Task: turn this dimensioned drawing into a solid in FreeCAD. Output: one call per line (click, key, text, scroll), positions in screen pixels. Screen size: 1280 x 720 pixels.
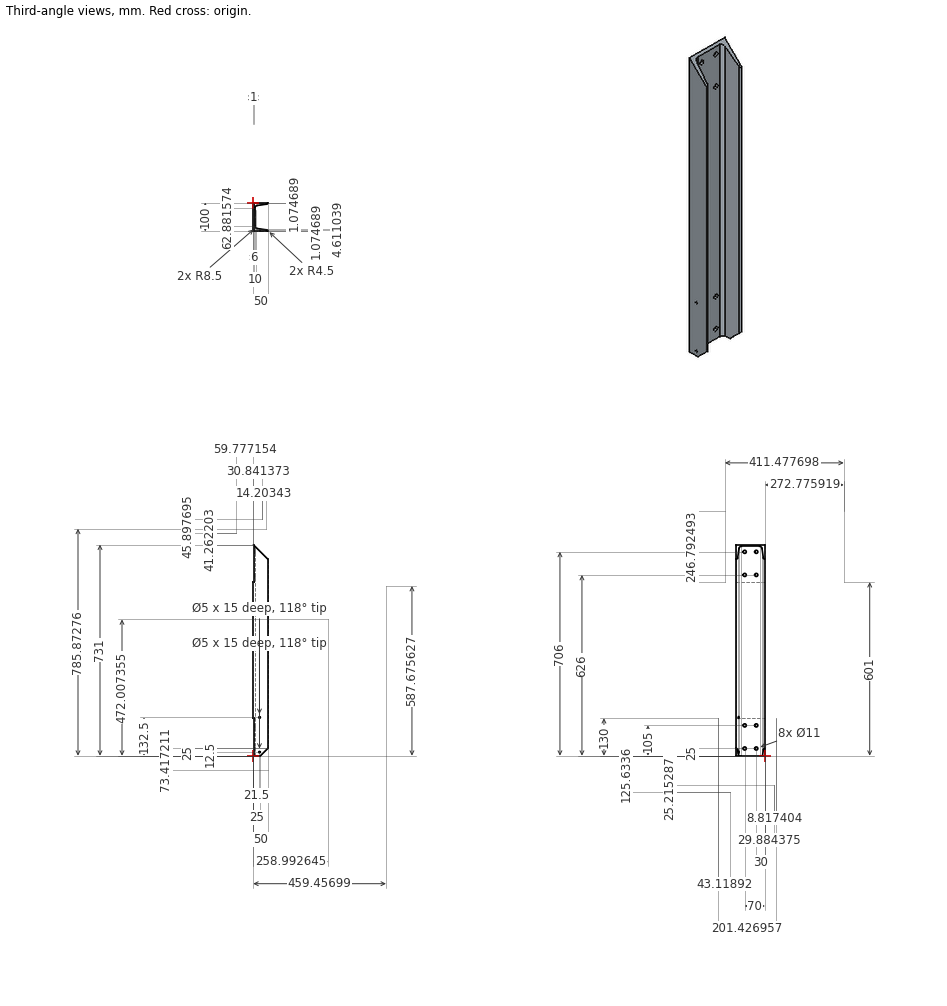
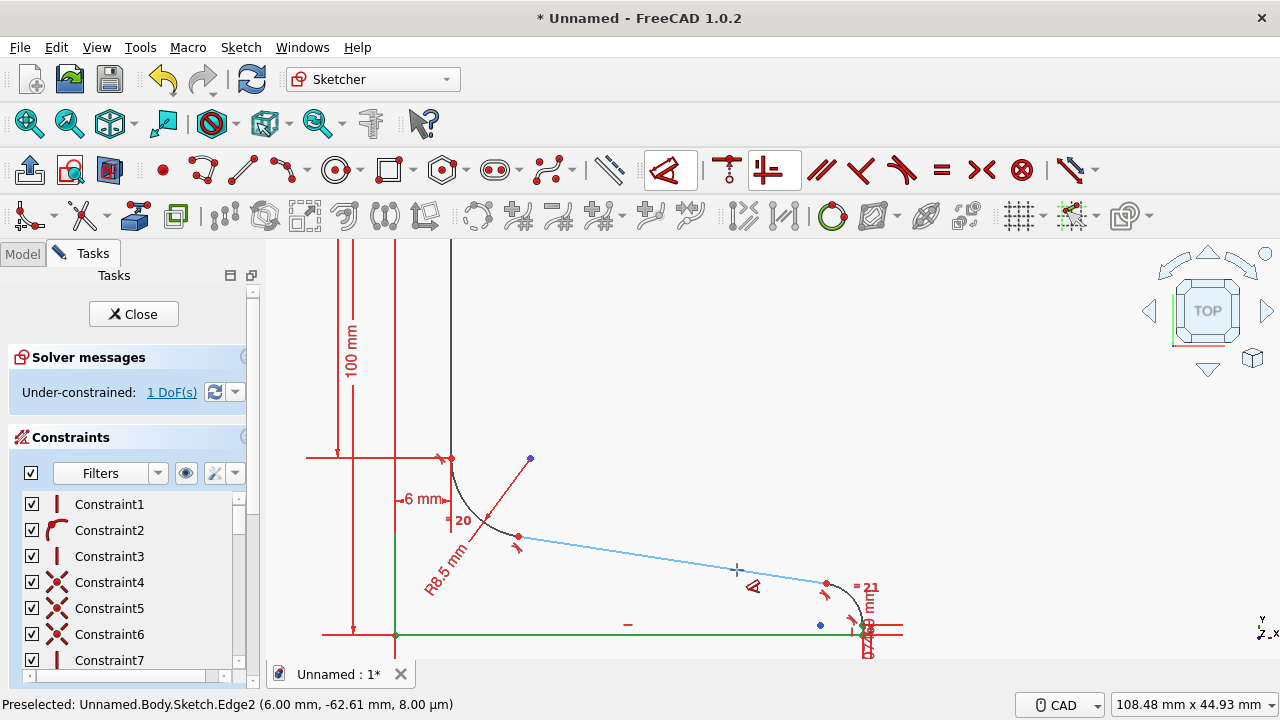
click(734, 570)
click(861, 560)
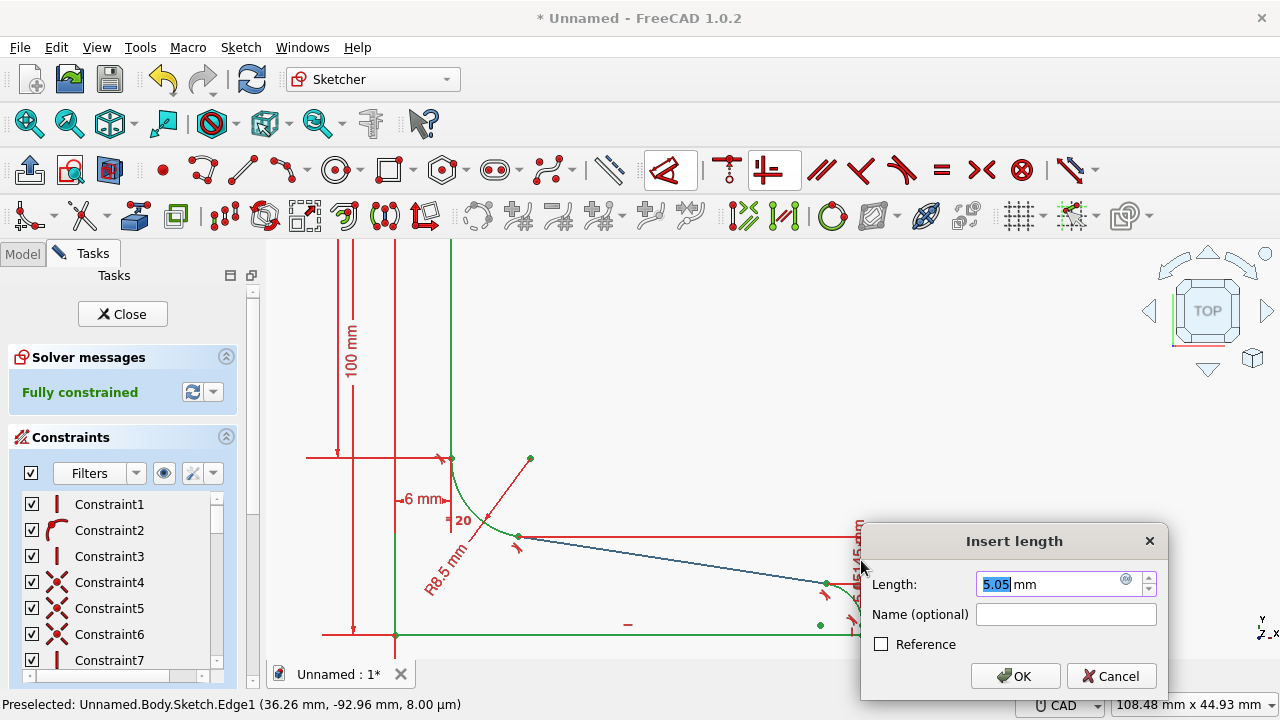
text(4.611039)
key(Return)
key(Escape)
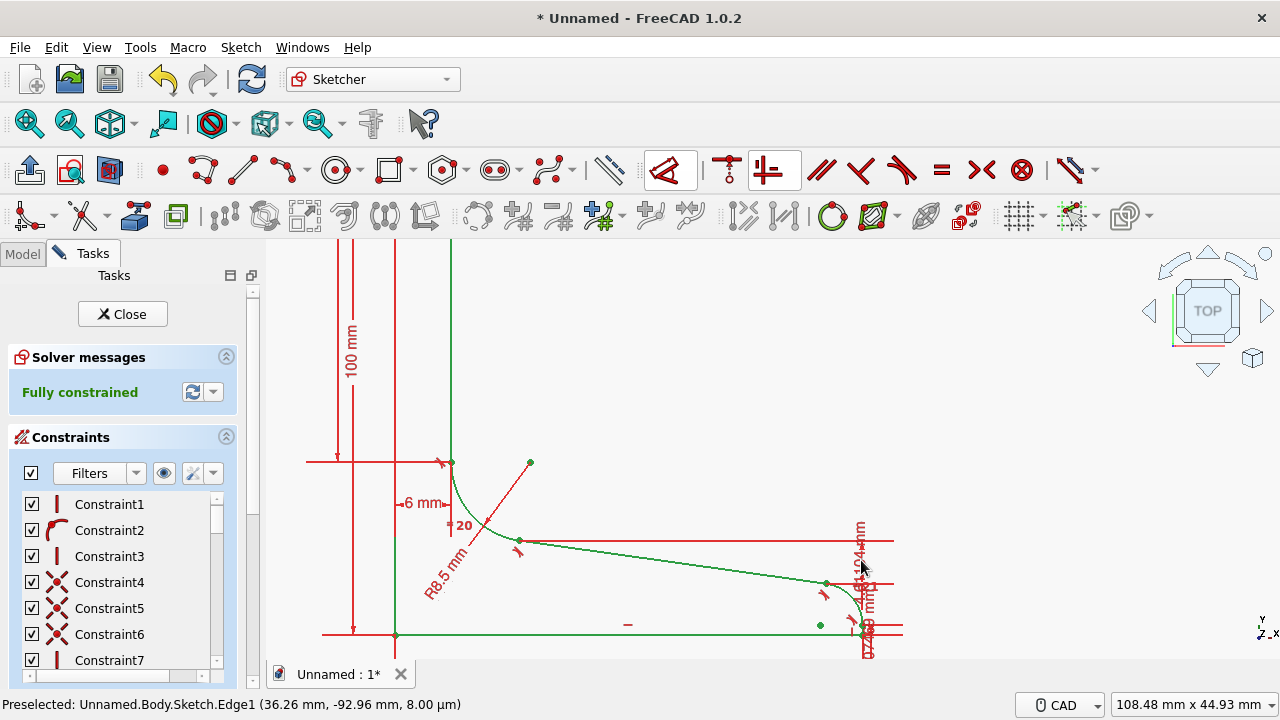
click(123, 314)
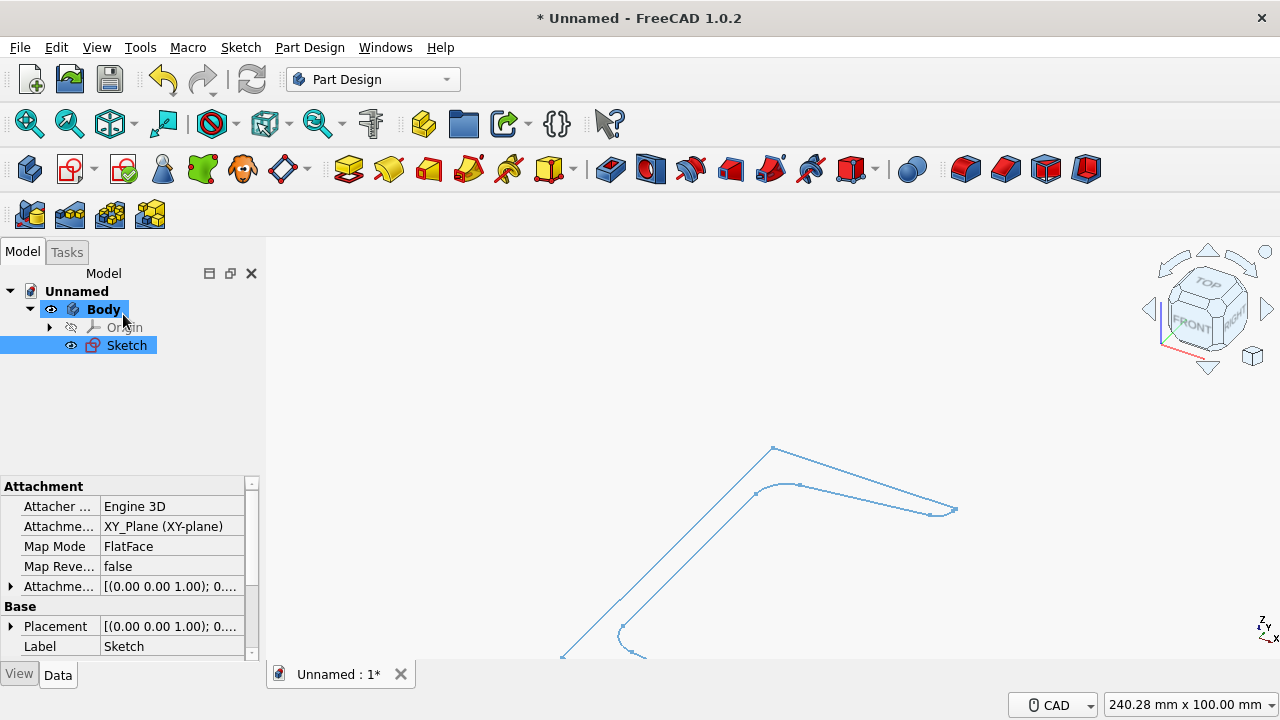
click(350, 170)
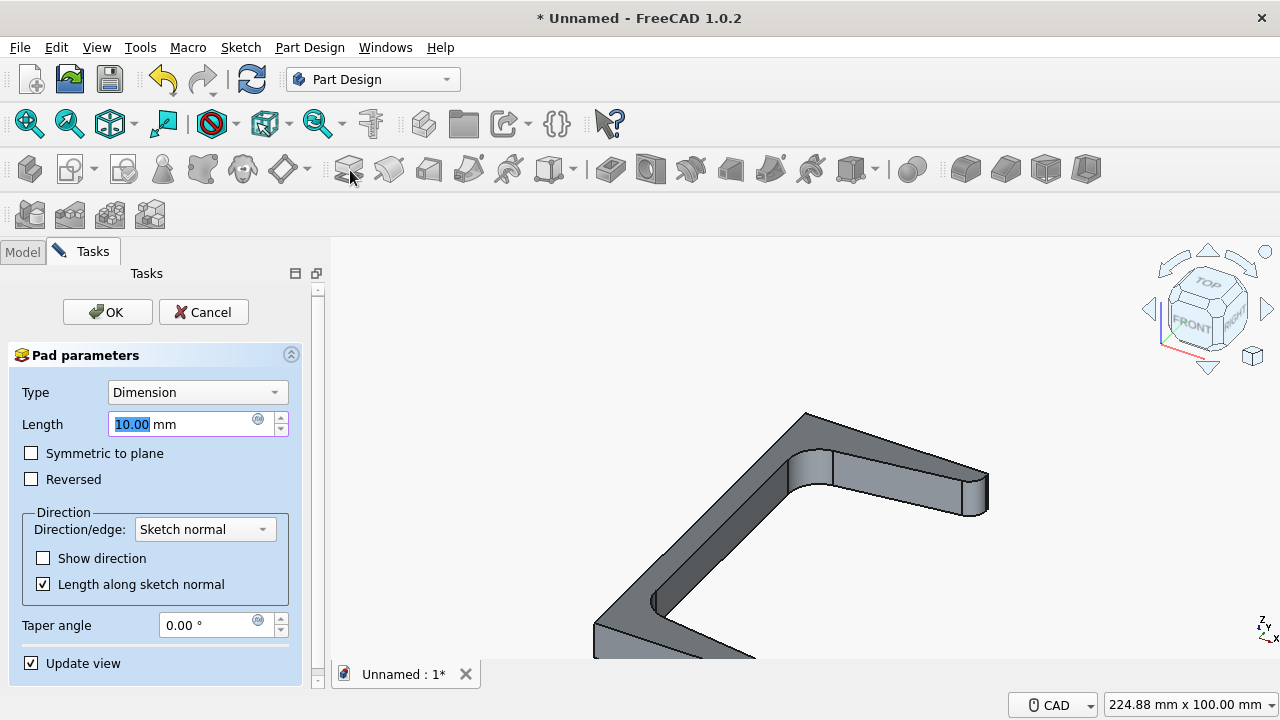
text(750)
key(Tab)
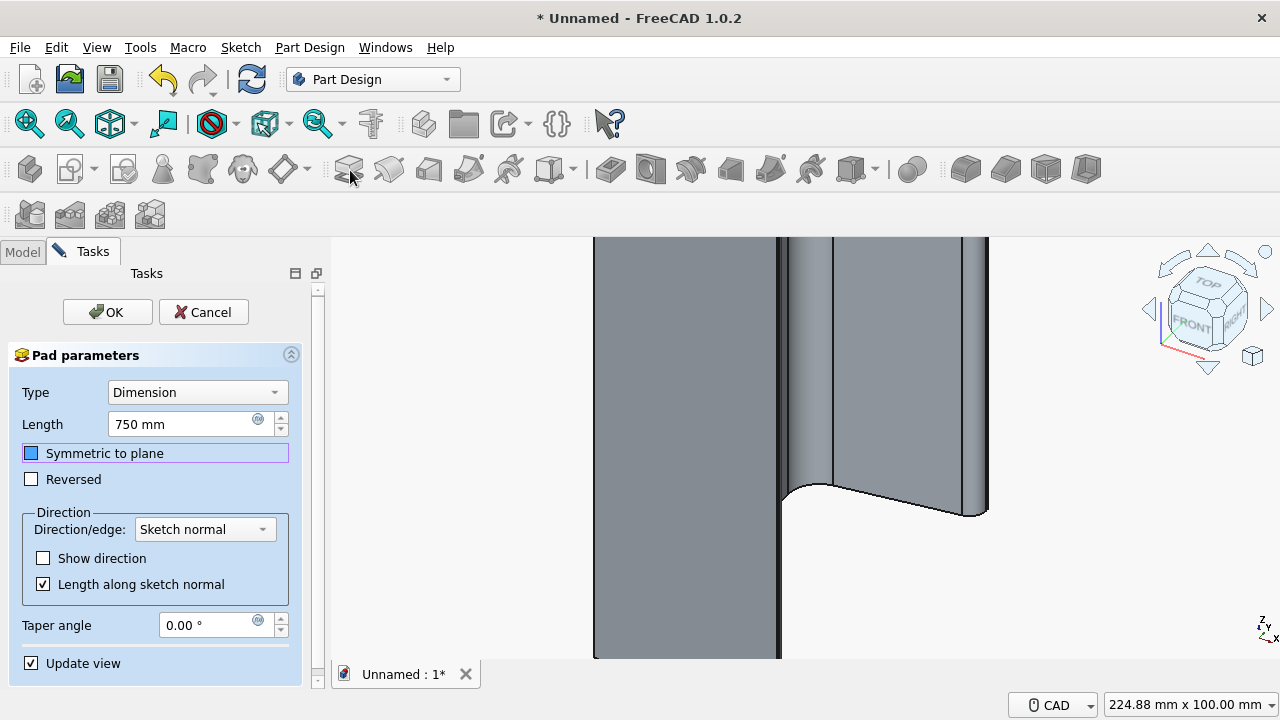
click(108, 312)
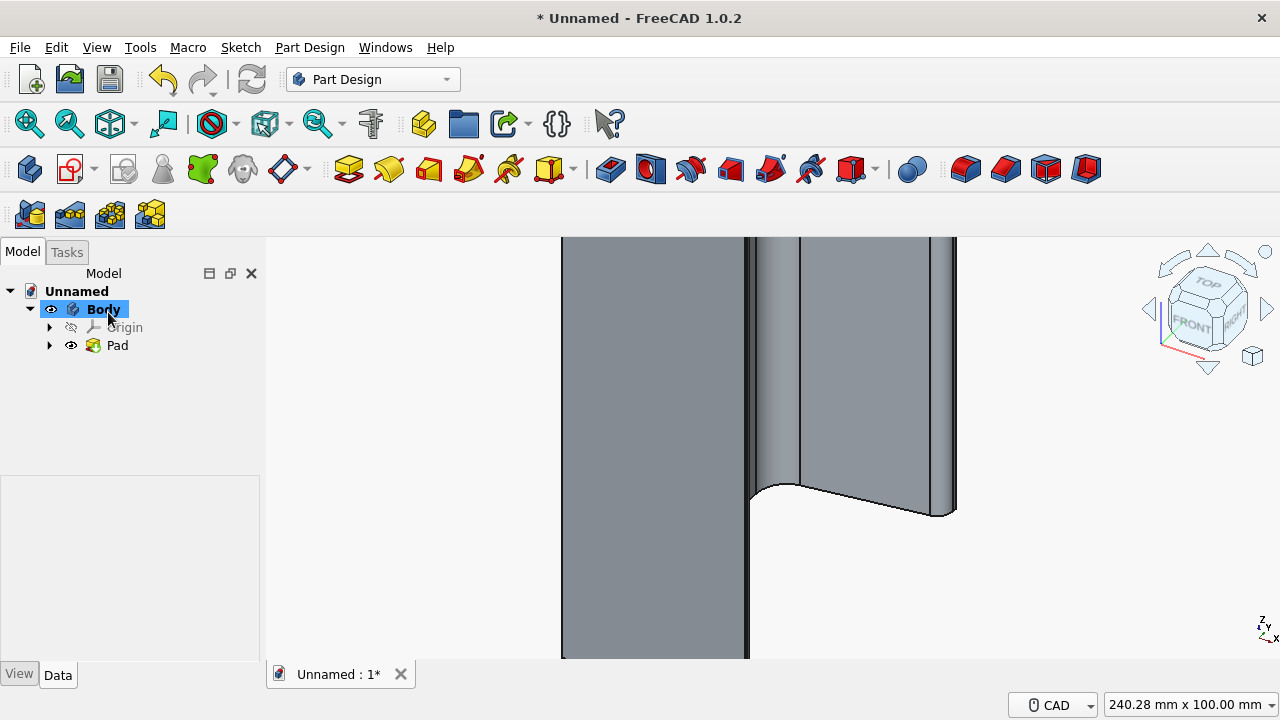
click(30, 124)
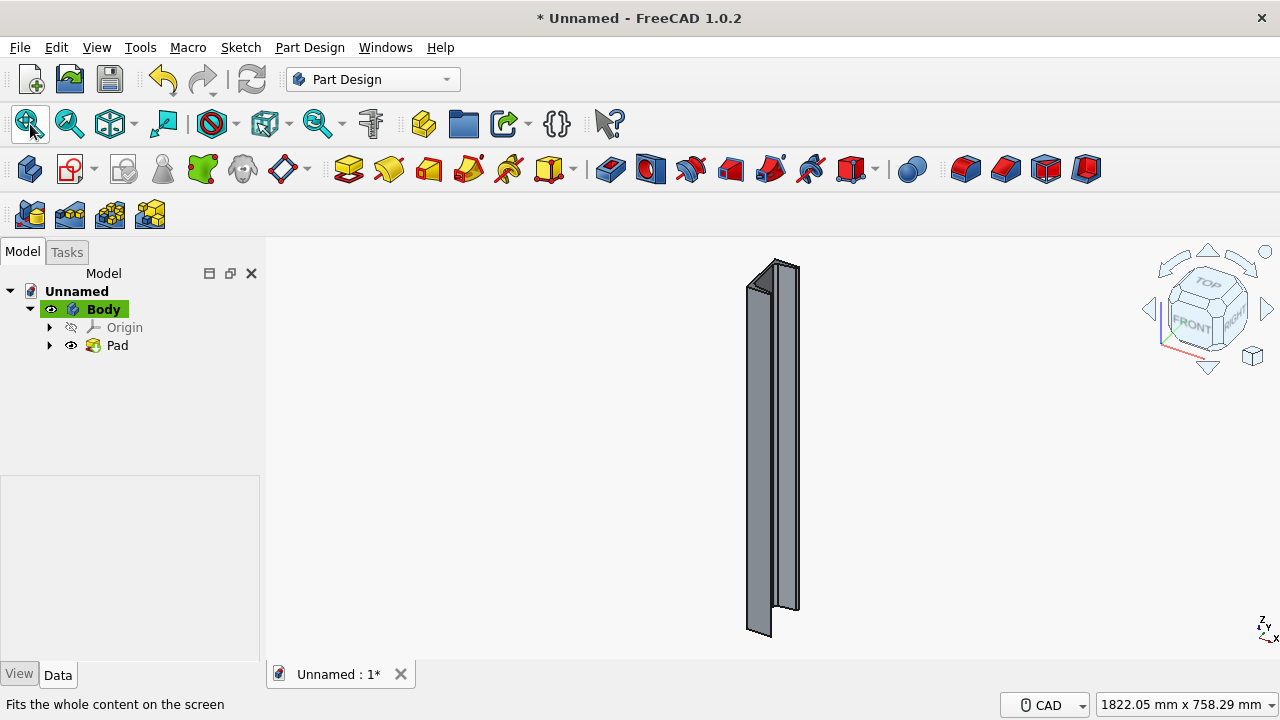
click(70, 170)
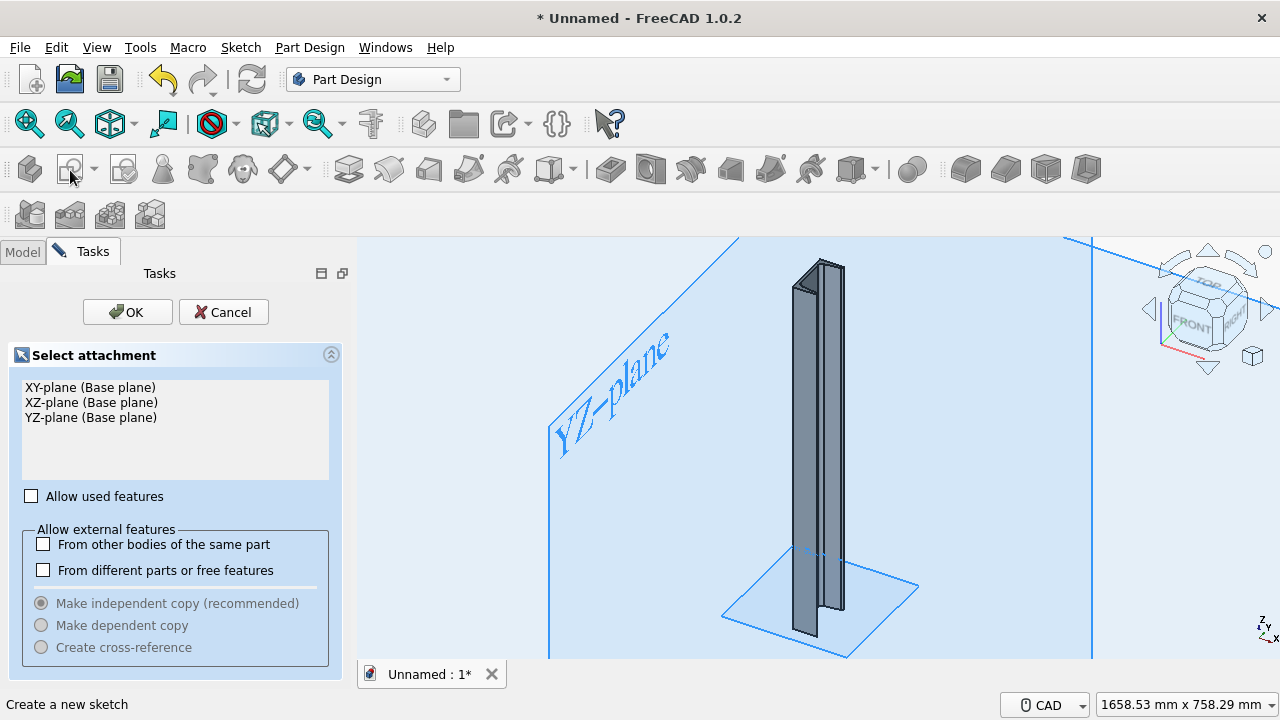
click(82, 402)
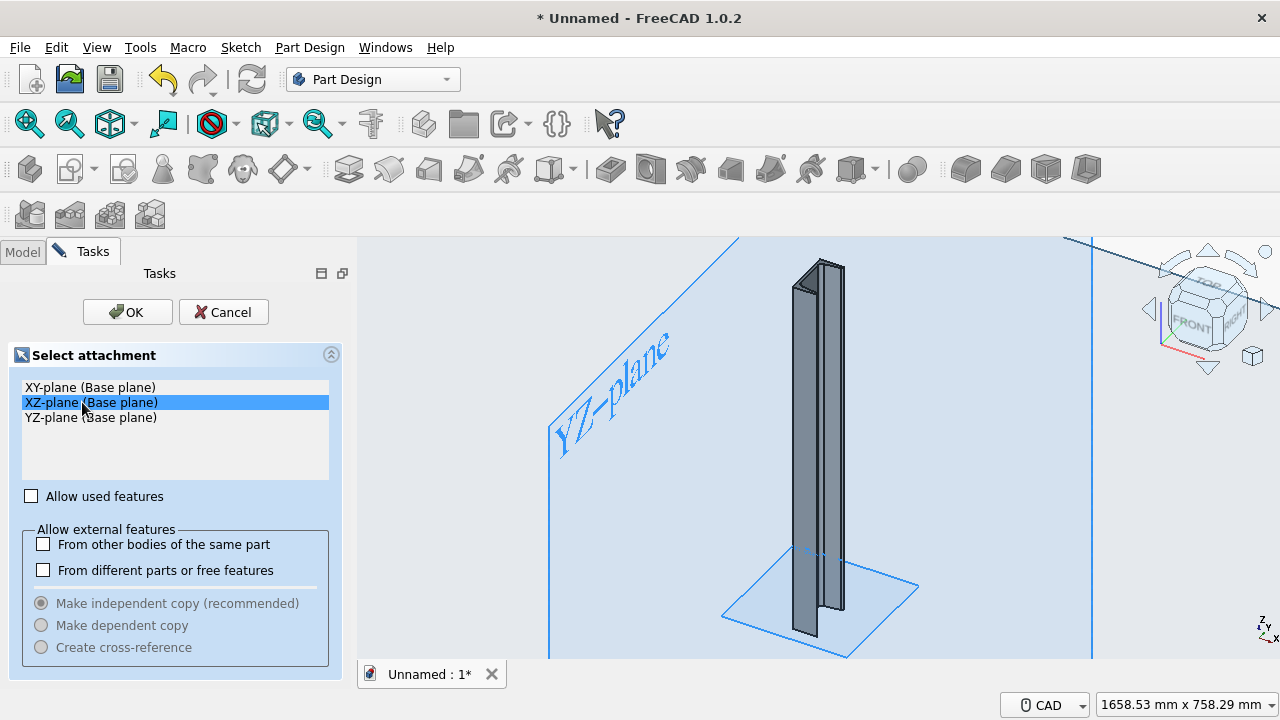
click(128, 312)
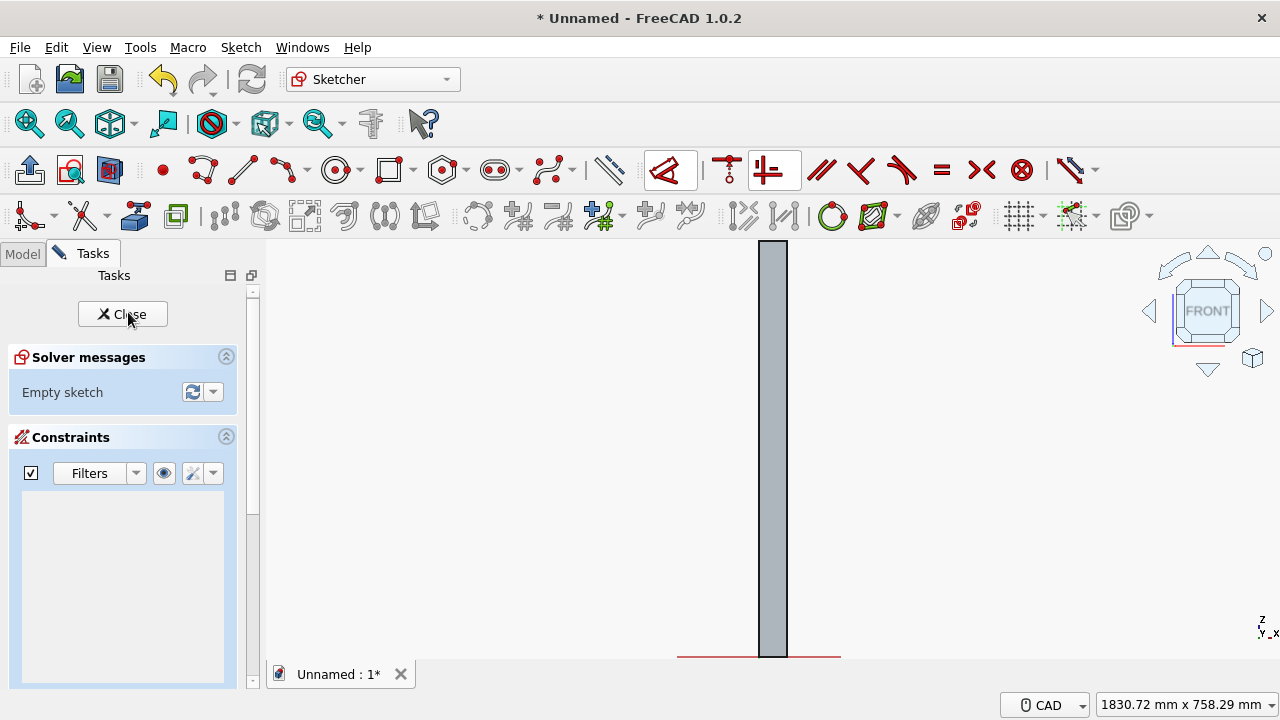
key(q)
key(s)